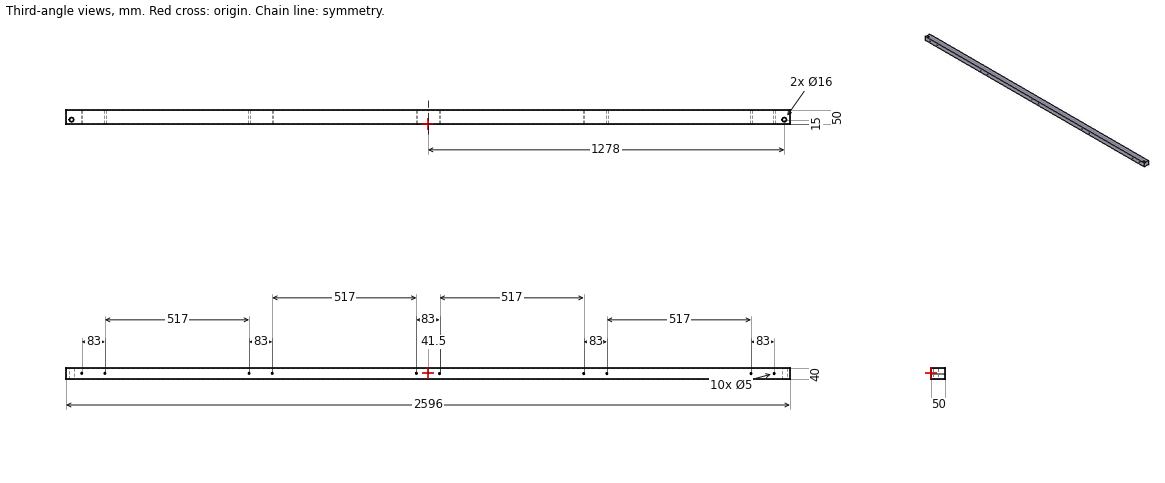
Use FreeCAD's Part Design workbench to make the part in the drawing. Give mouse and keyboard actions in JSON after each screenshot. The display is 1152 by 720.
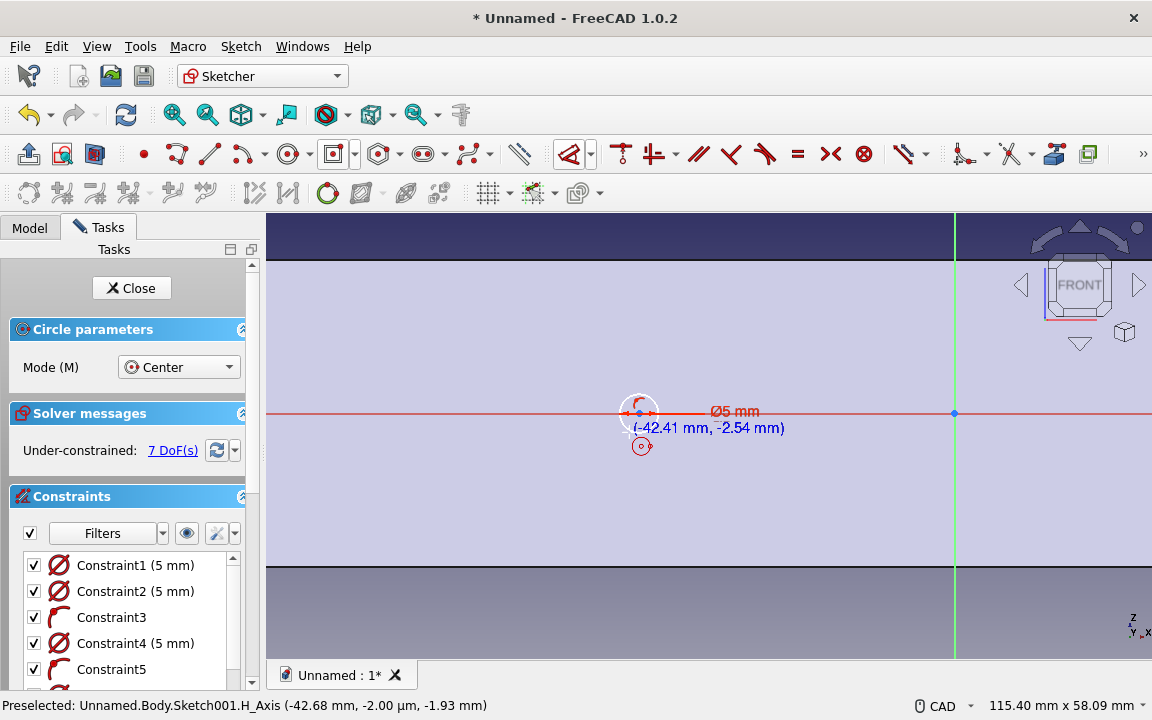
{"action": "scroll", "coordinate": [630, 437], "scroll_direction": "down", "scroll_amount": 17}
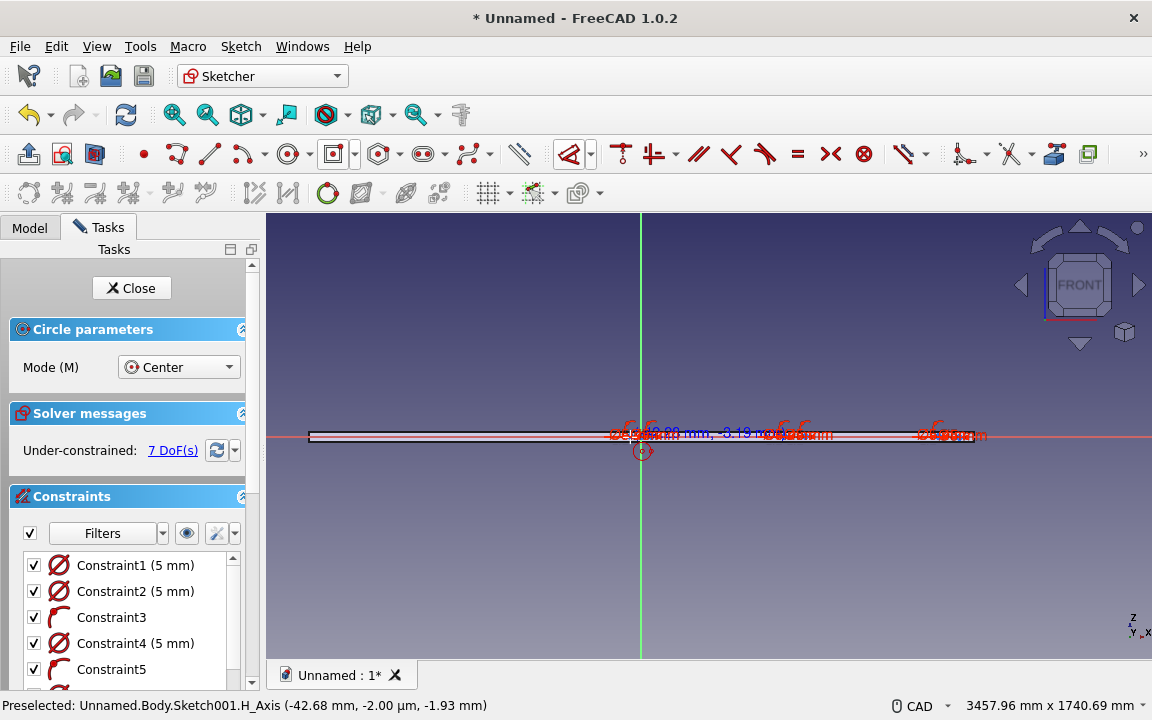
{"action": "scroll", "coordinate": [498, 437], "scroll_direction": "up", "scroll_amount": 18}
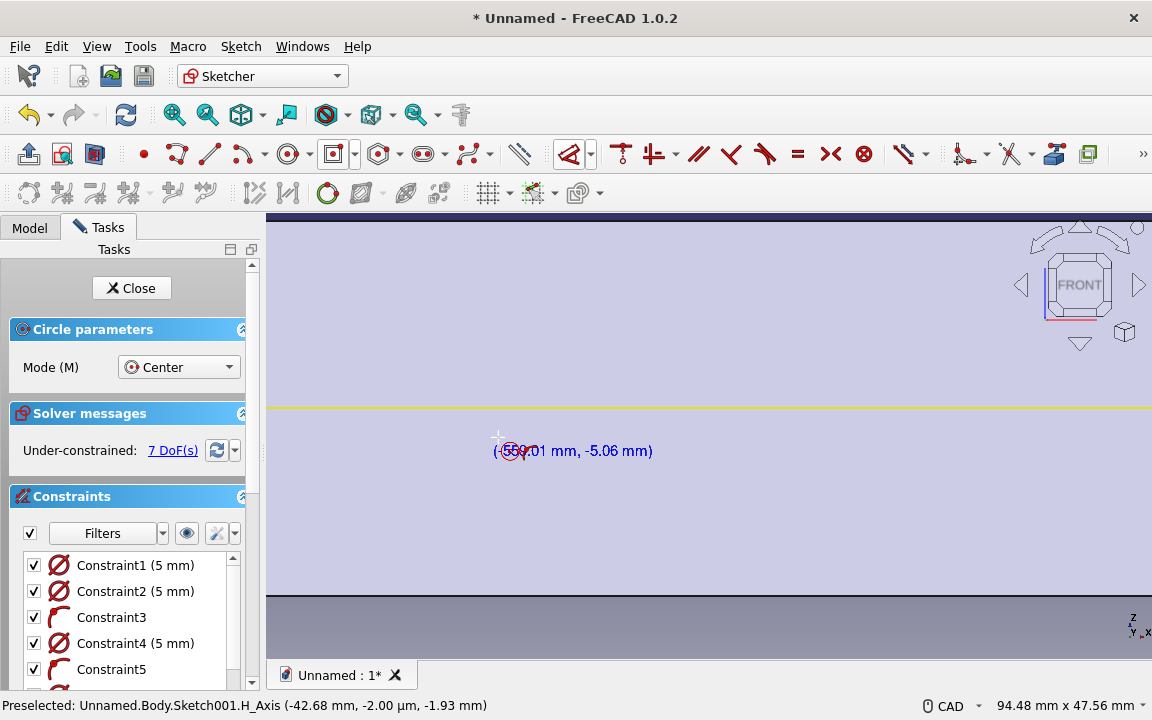
{"action": "scroll", "coordinate": [498, 437], "scroll_direction": "down", "scroll_amount": 18}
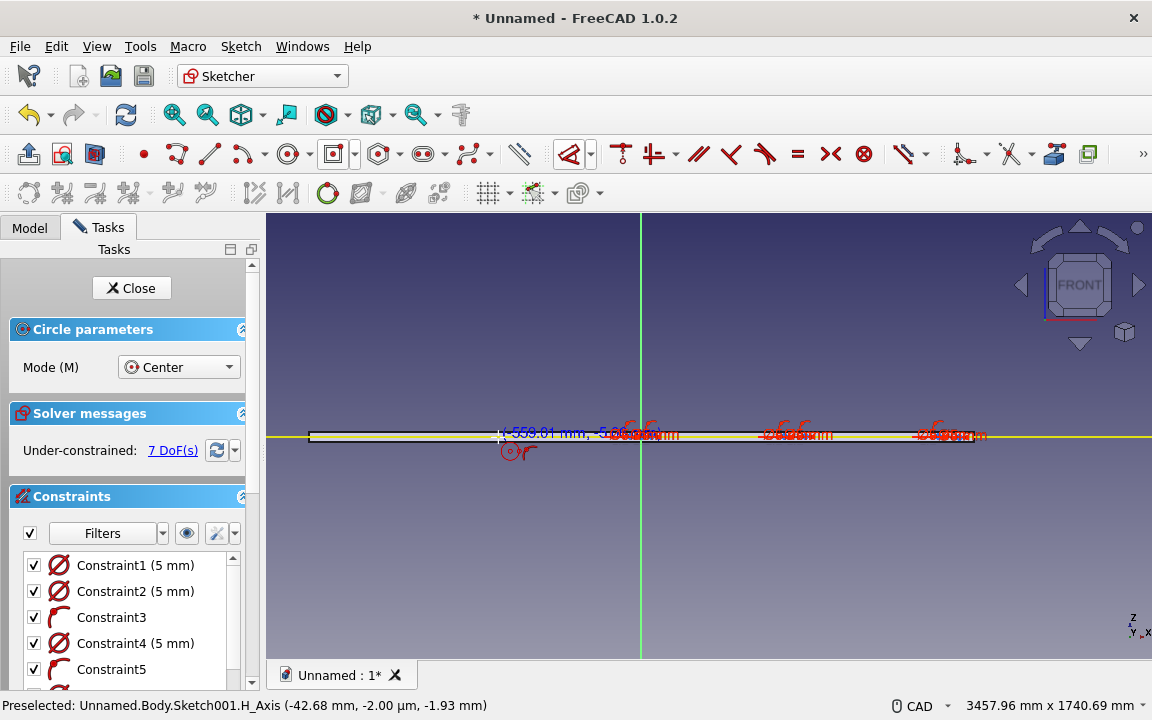
{"action": "left_click", "coordinate": [498, 437]}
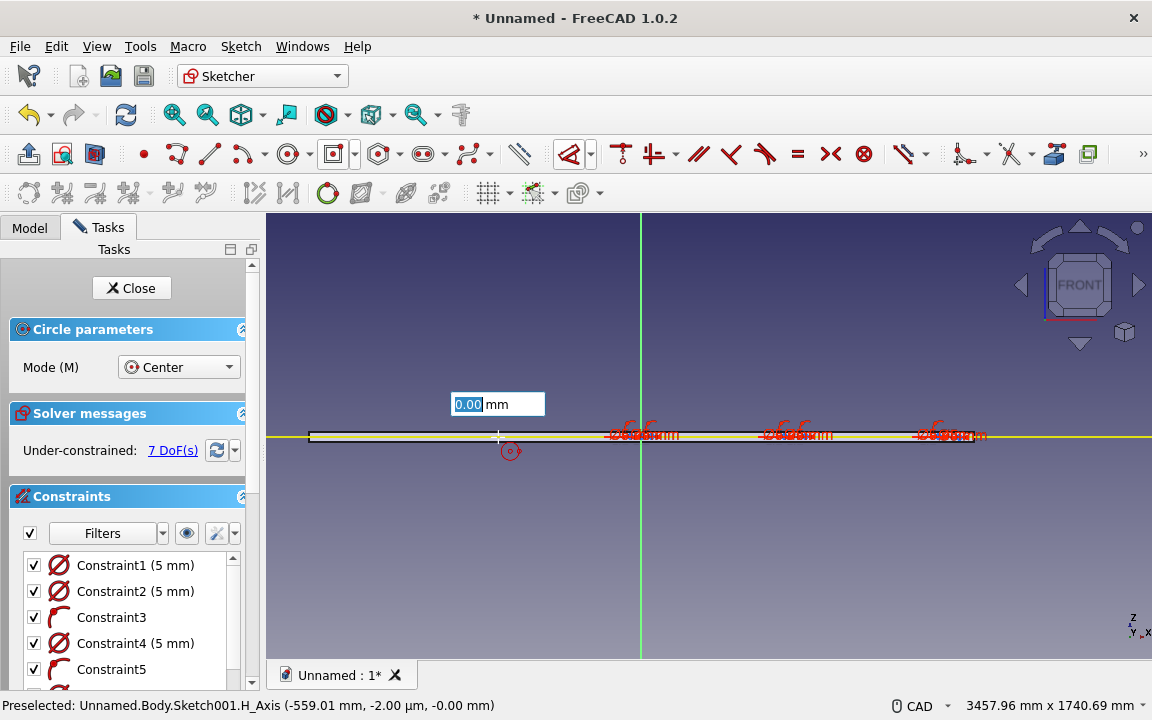
{"action": "scroll", "coordinate": [498, 437], "scroll_direction": "up", "scroll_amount": 17}
{"action": "mouse_move", "coordinate": [488, 432]}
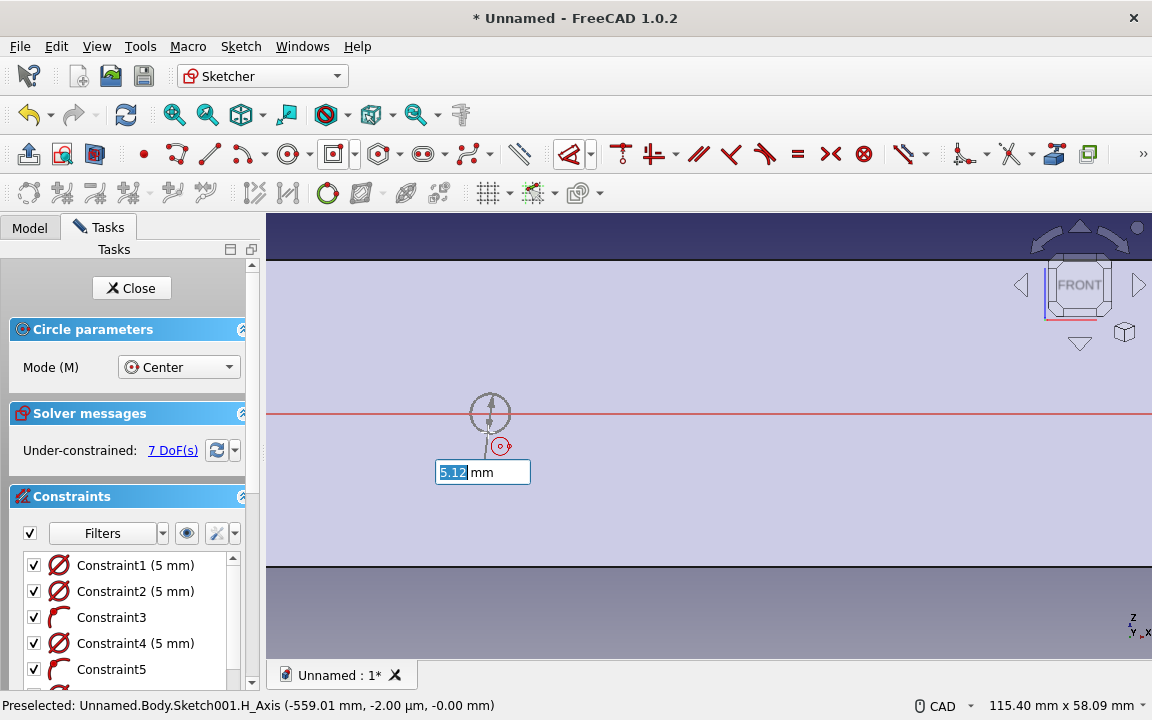
{"action": "type", "text": "5"}
{"action": "key", "text": "Return"}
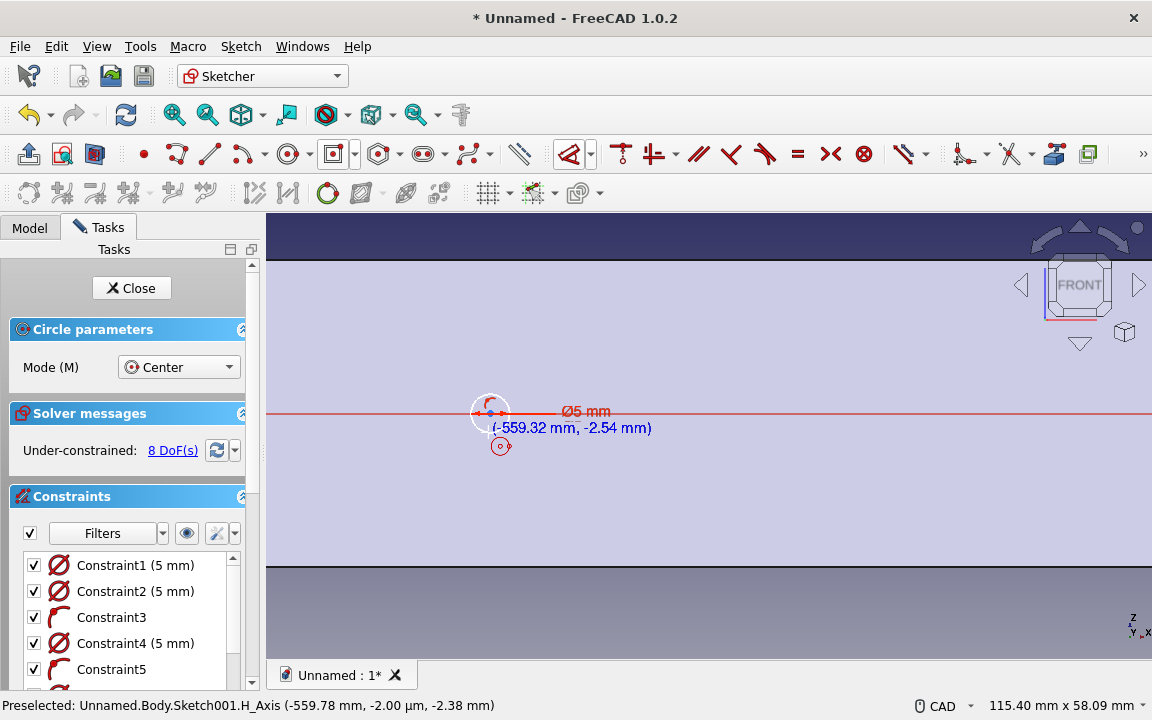
{"action": "scroll", "coordinate": [498, 437], "scroll_direction": "down", "scroll_amount": 17}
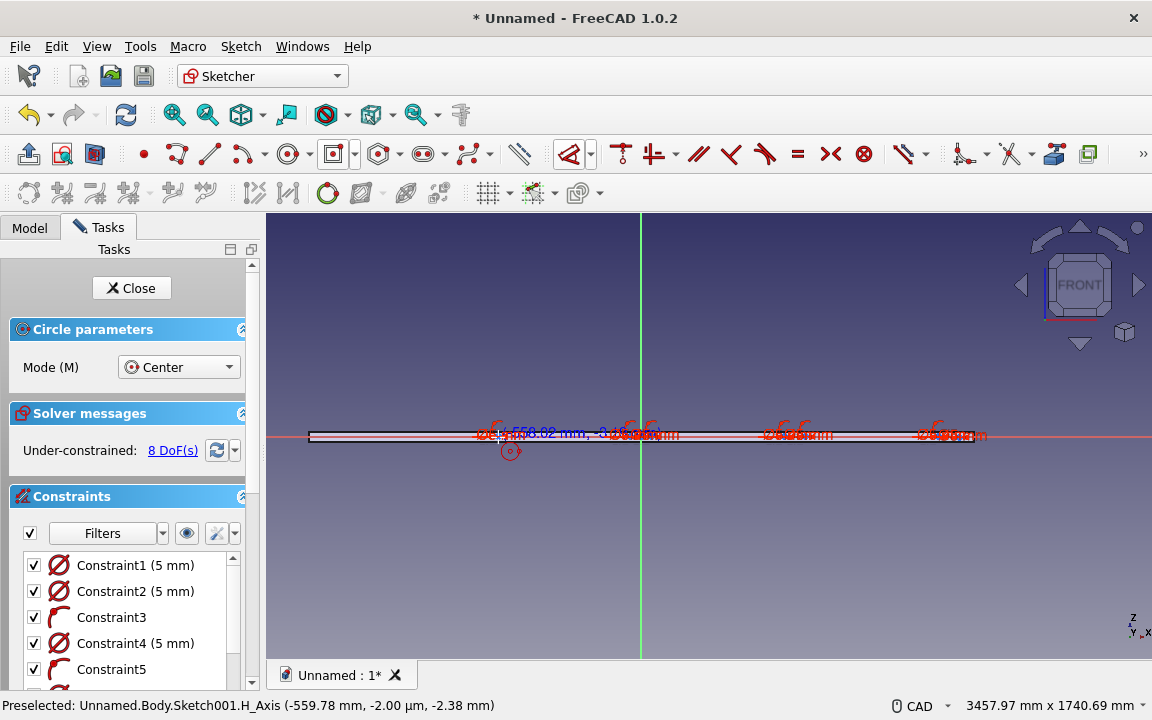
{"action": "scroll", "coordinate": [477, 437], "scroll_direction": "up", "scroll_amount": 18}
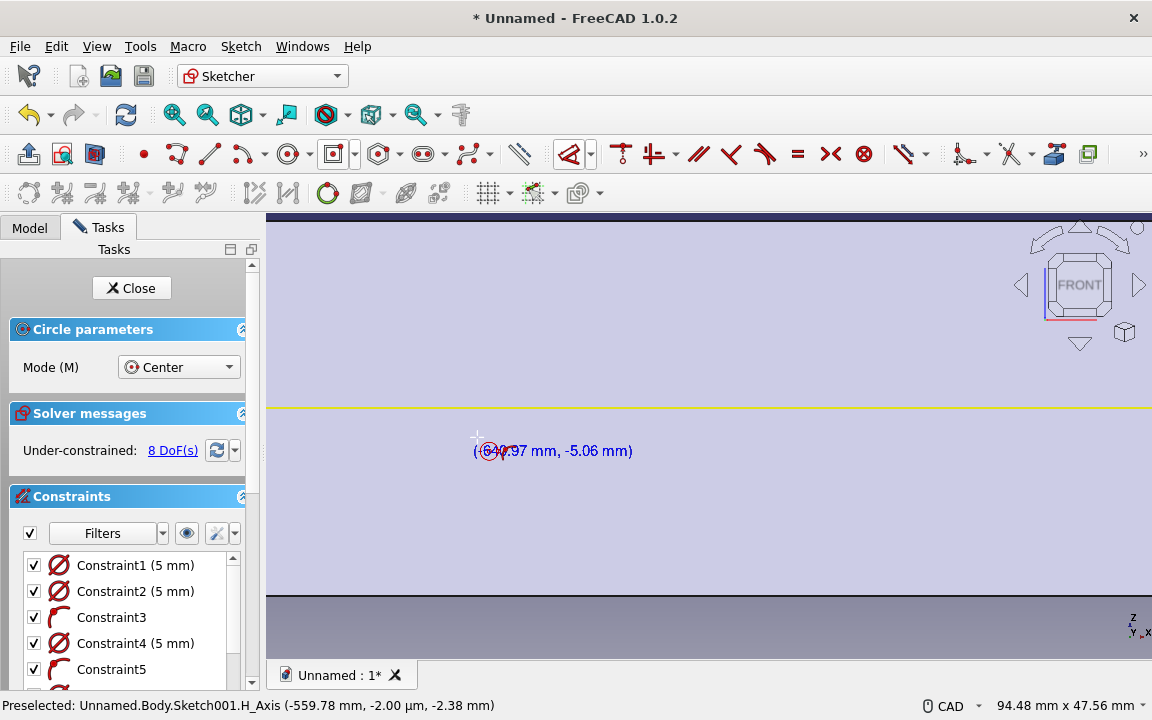
{"action": "scroll", "coordinate": [476, 437], "scroll_direction": "down", "scroll_amount": 18}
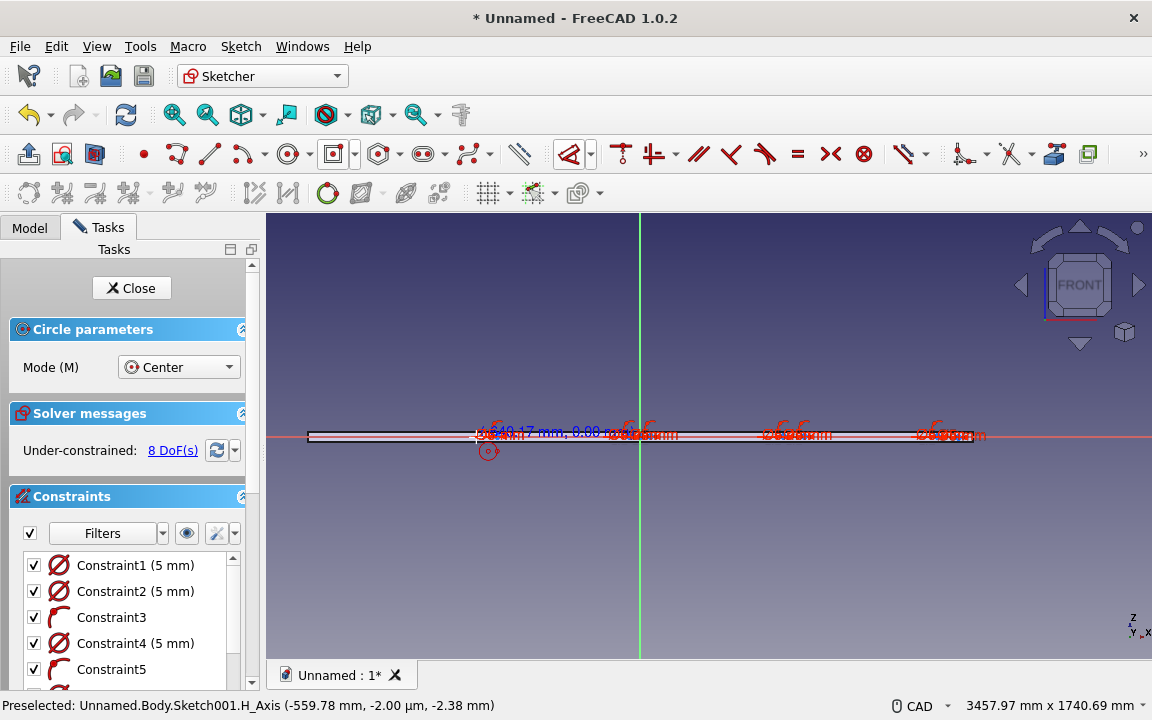
{"action": "left_click", "coordinate": [476, 437]}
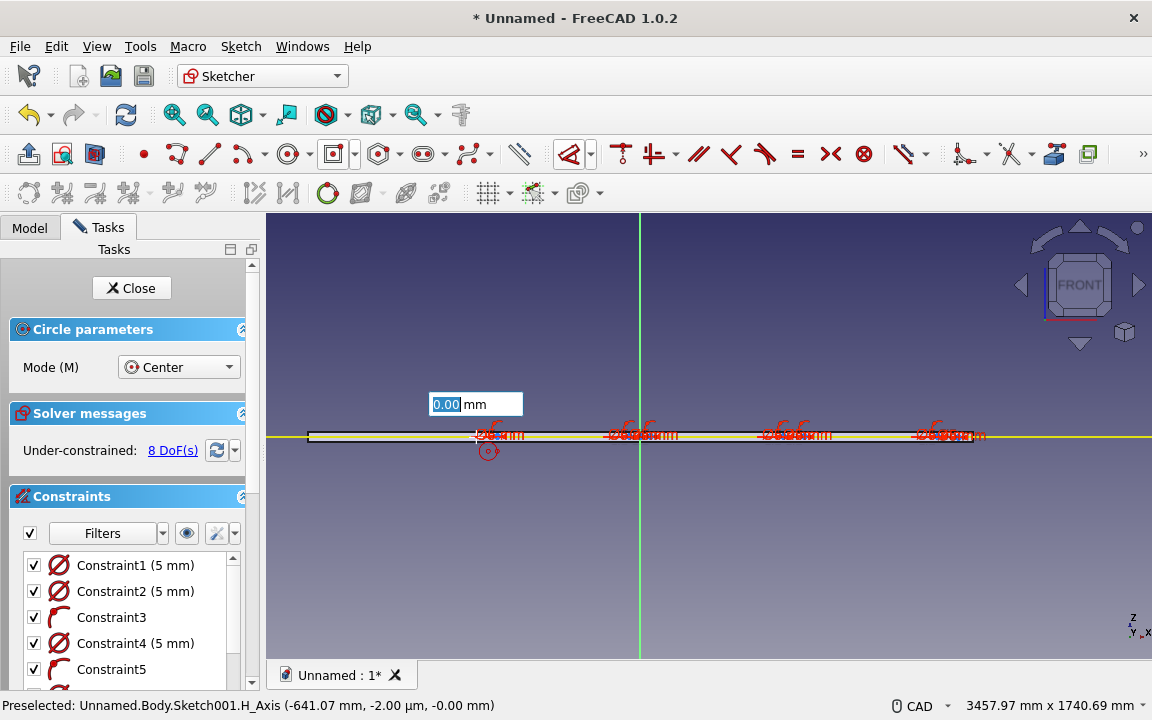
{"action": "scroll", "coordinate": [476, 437], "scroll_direction": "up", "scroll_amount": 17}
{"action": "mouse_move", "coordinate": [459, 432]}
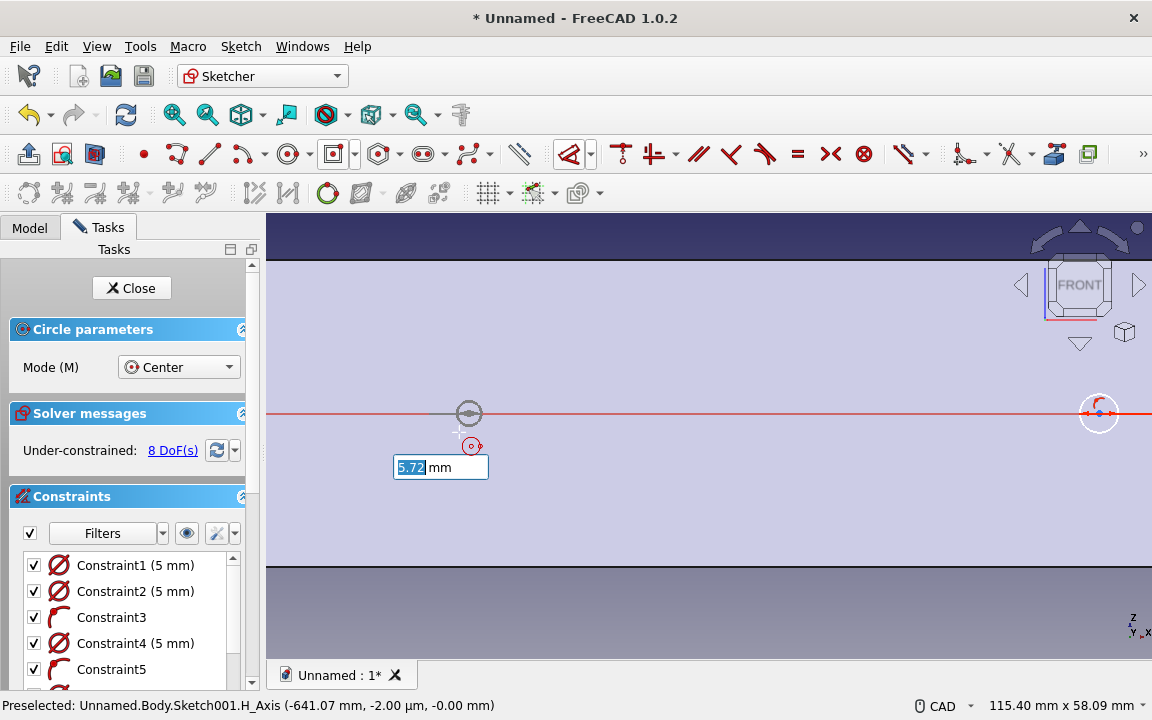
{"action": "type", "text": "5"}
{"action": "key", "text": "Return"}